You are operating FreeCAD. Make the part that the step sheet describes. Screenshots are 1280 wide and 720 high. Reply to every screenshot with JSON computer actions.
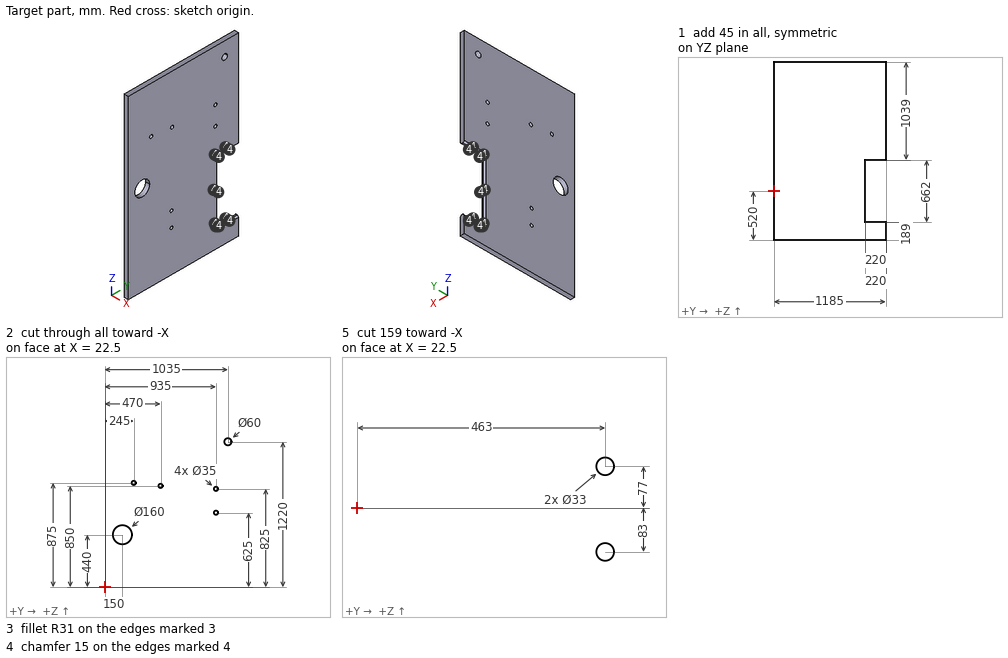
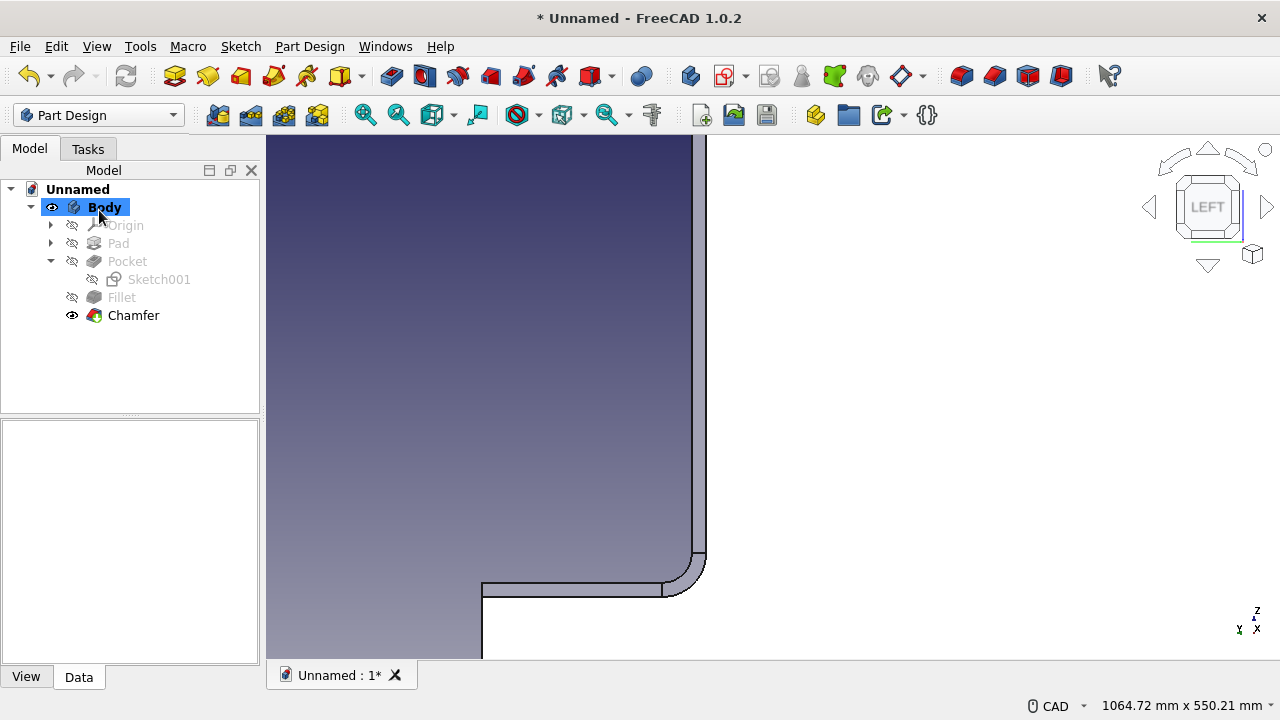
{"action": "left_click", "coordinate": [366, 116]}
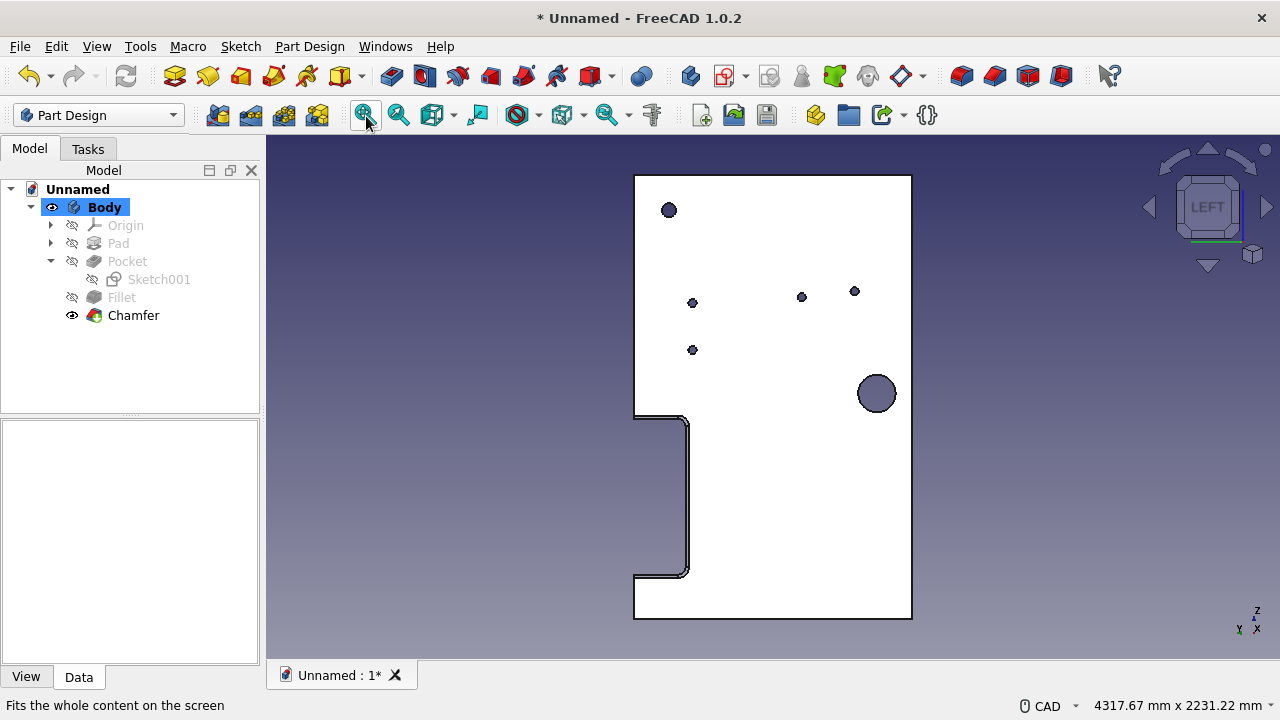
{"action": "key", "text": "0"}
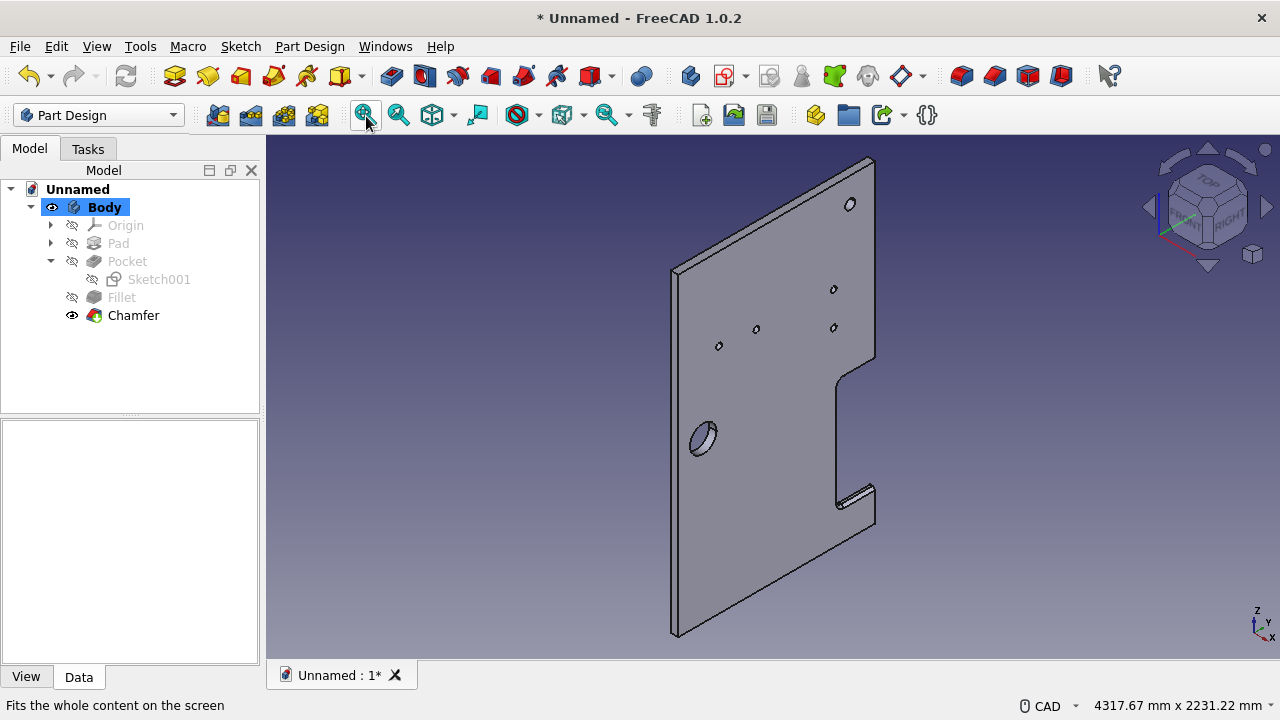
{"action": "left_click", "coordinate": [749, 518]}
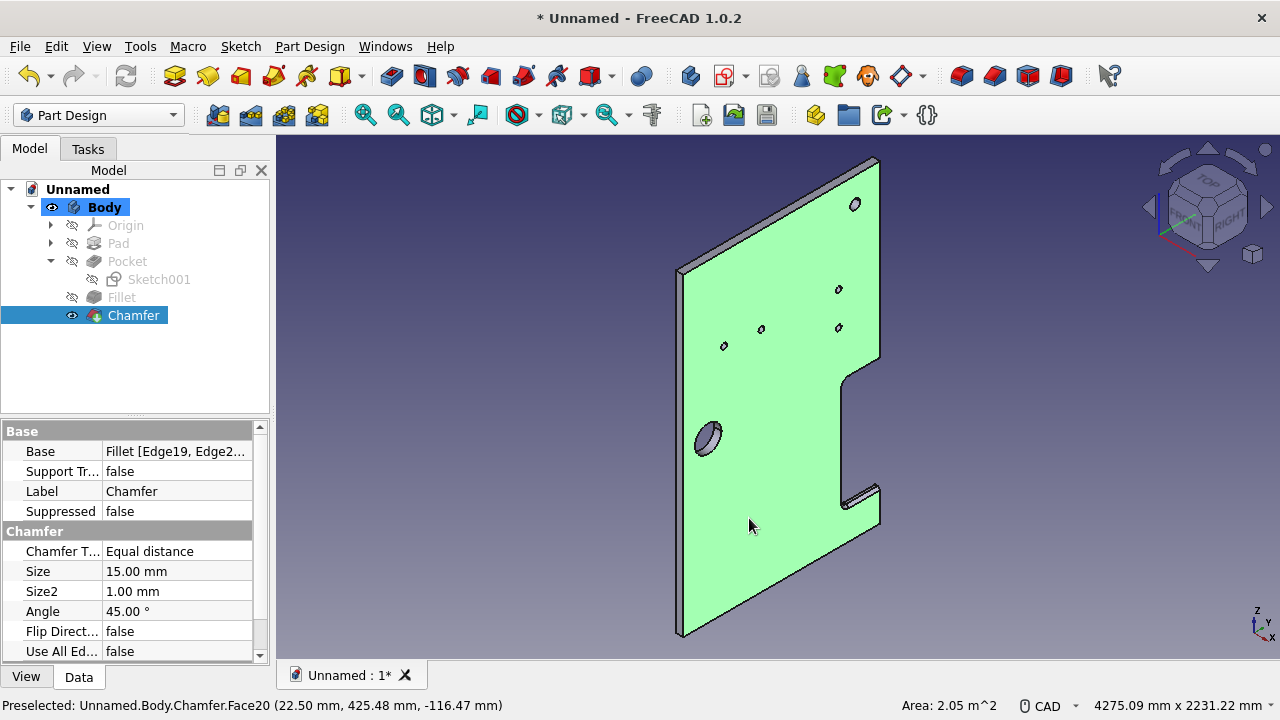
{"action": "left_click", "coordinate": [724, 76]}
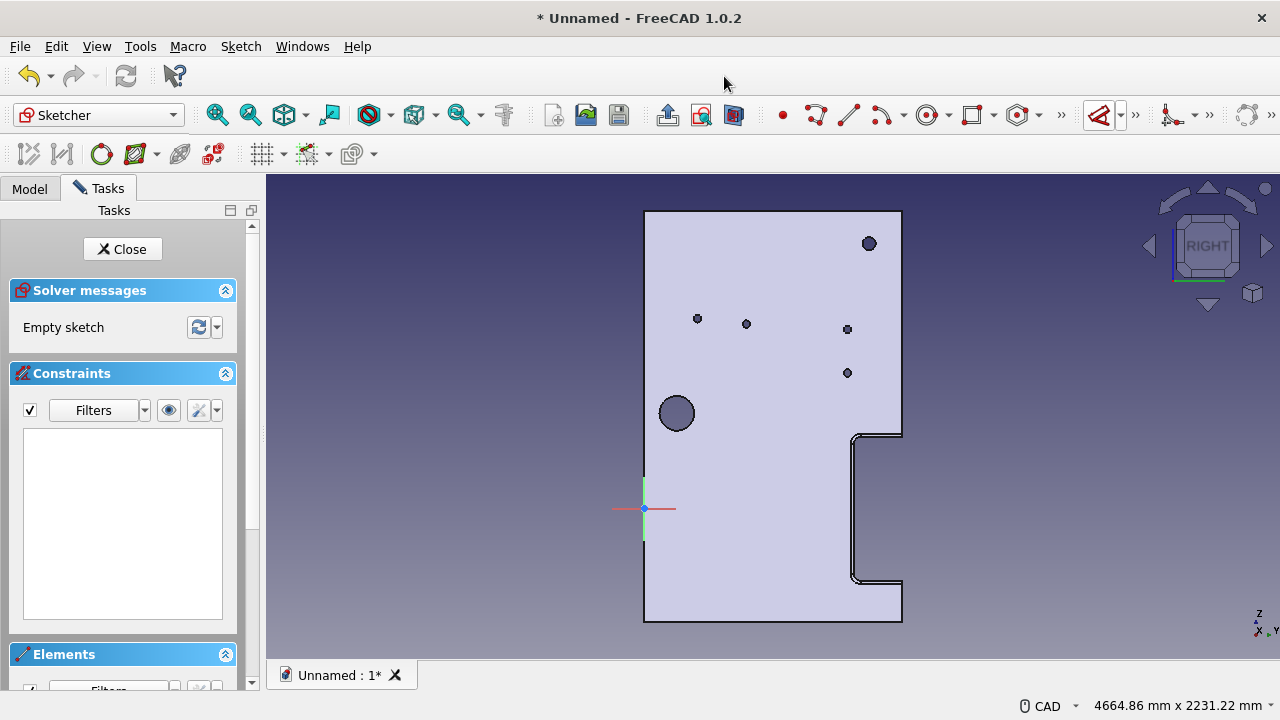
{"action": "scroll", "coordinate": [695, 528], "scroll_direction": "up", "scroll_amount": 9}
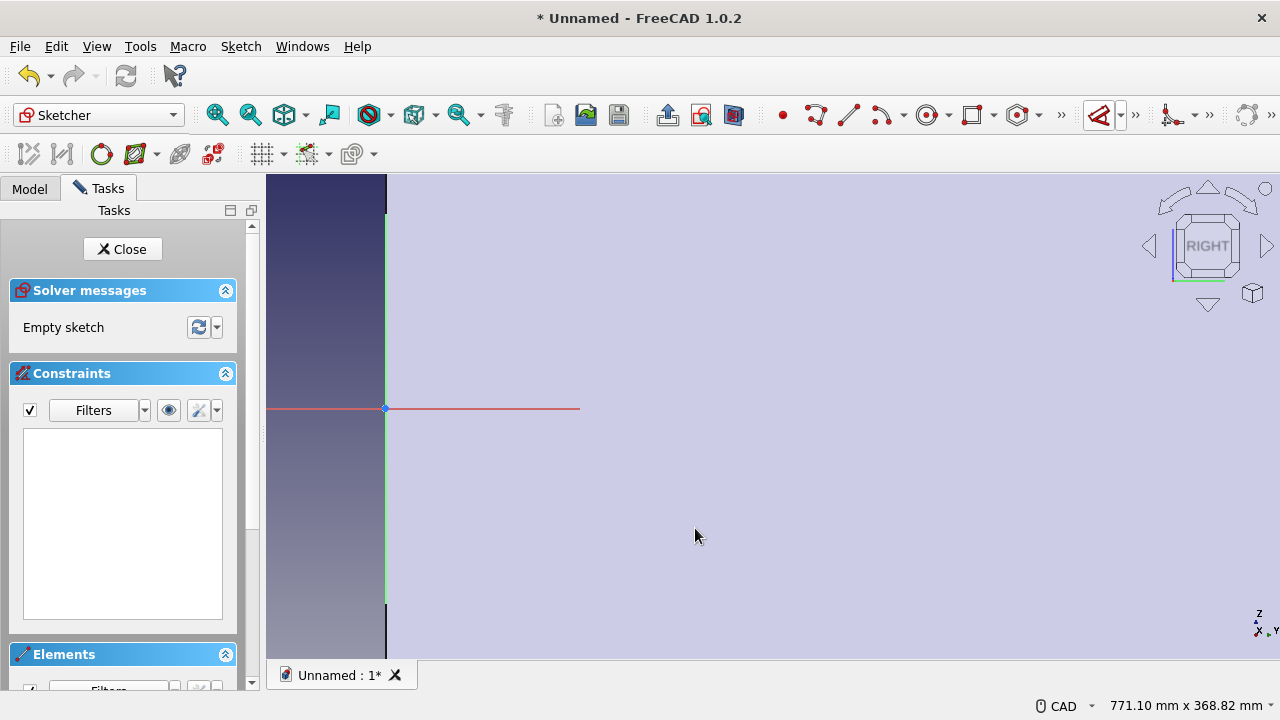
{"action": "left_click", "coordinate": [926, 116]}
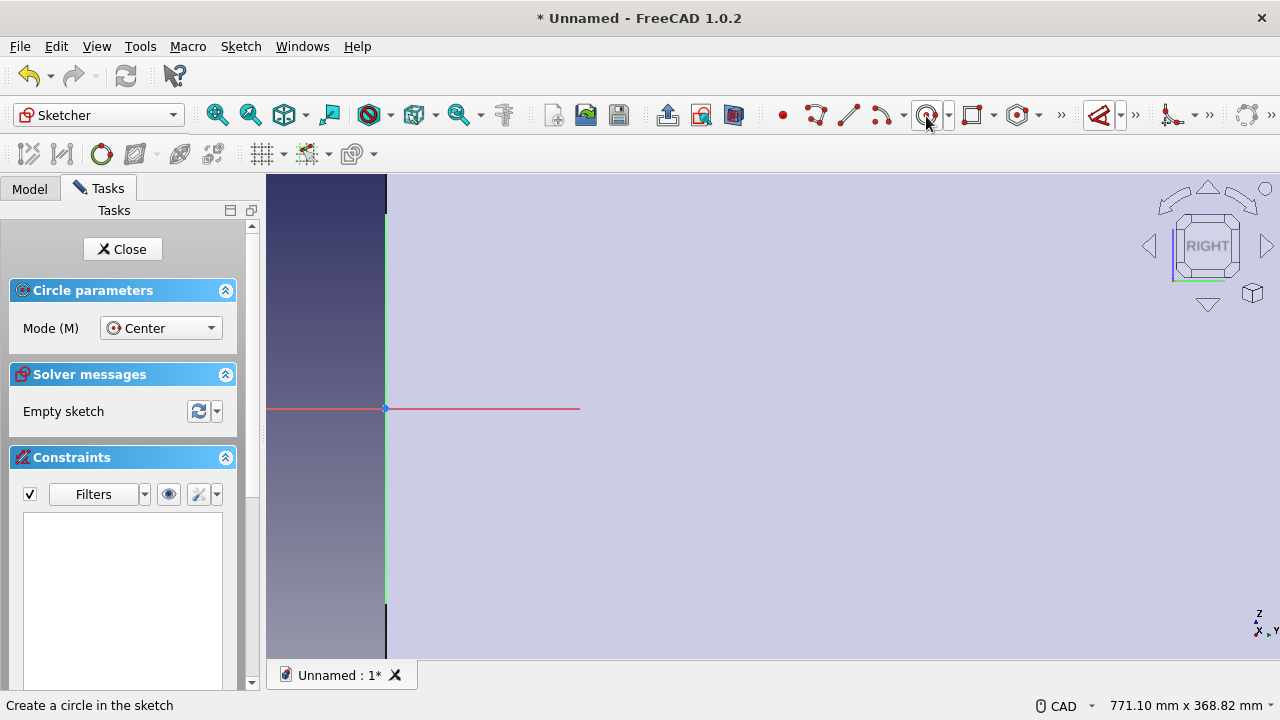
{"action": "left_click", "coordinate": [994, 307]}
{"action": "left_click", "coordinate": [1010, 292]}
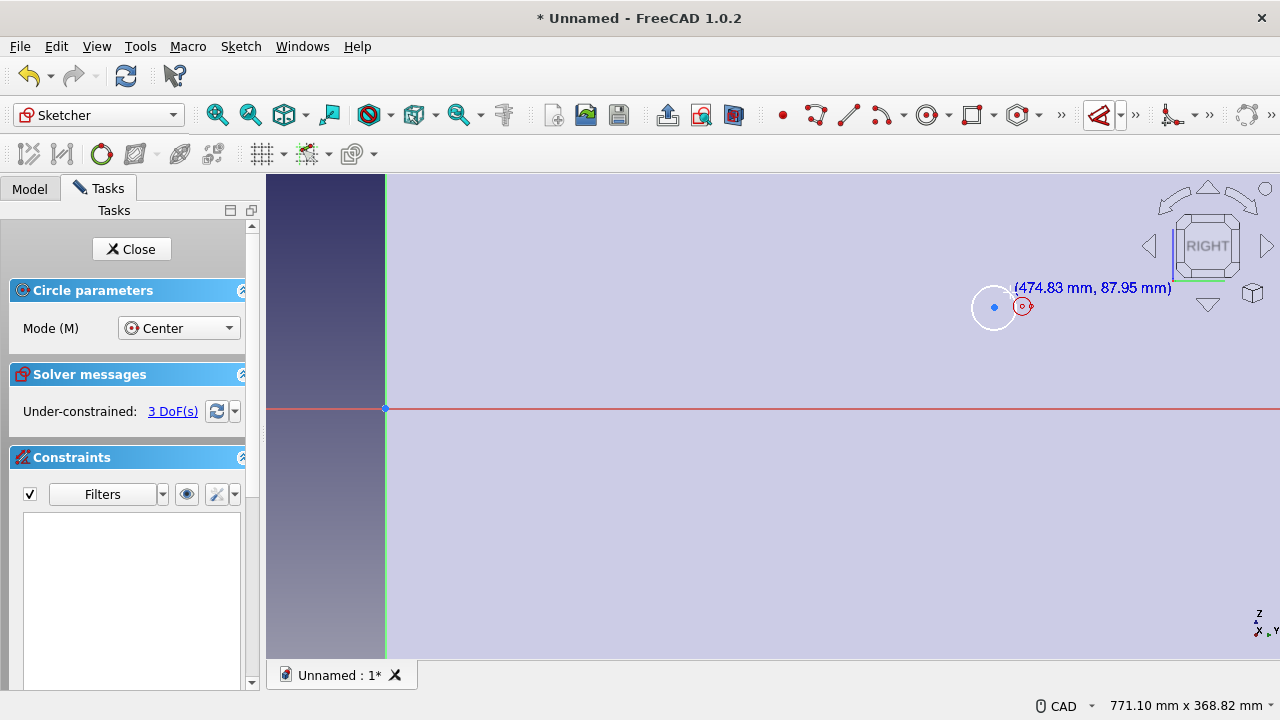
{"action": "left_click", "coordinate": [994, 518]}
{"action": "left_click", "coordinate": [1010, 502]}
{"action": "key", "text": "Escape"}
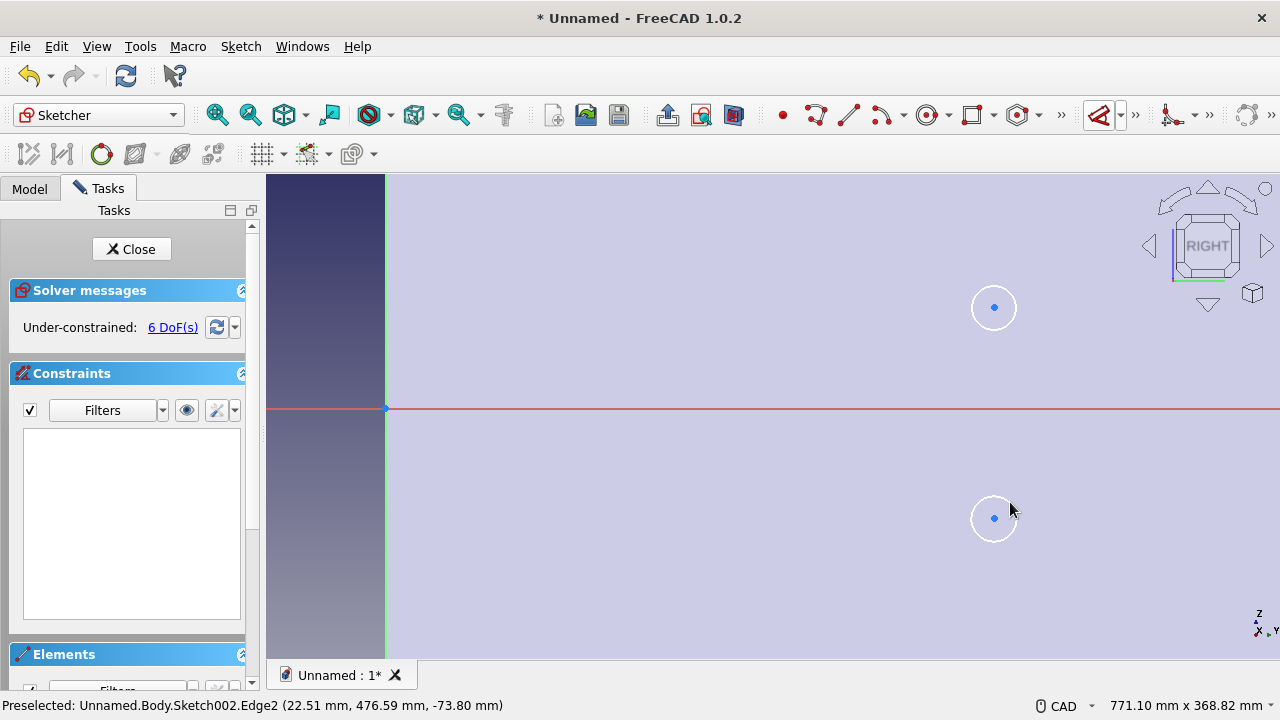
{"action": "left_click", "coordinate": [1009, 292]}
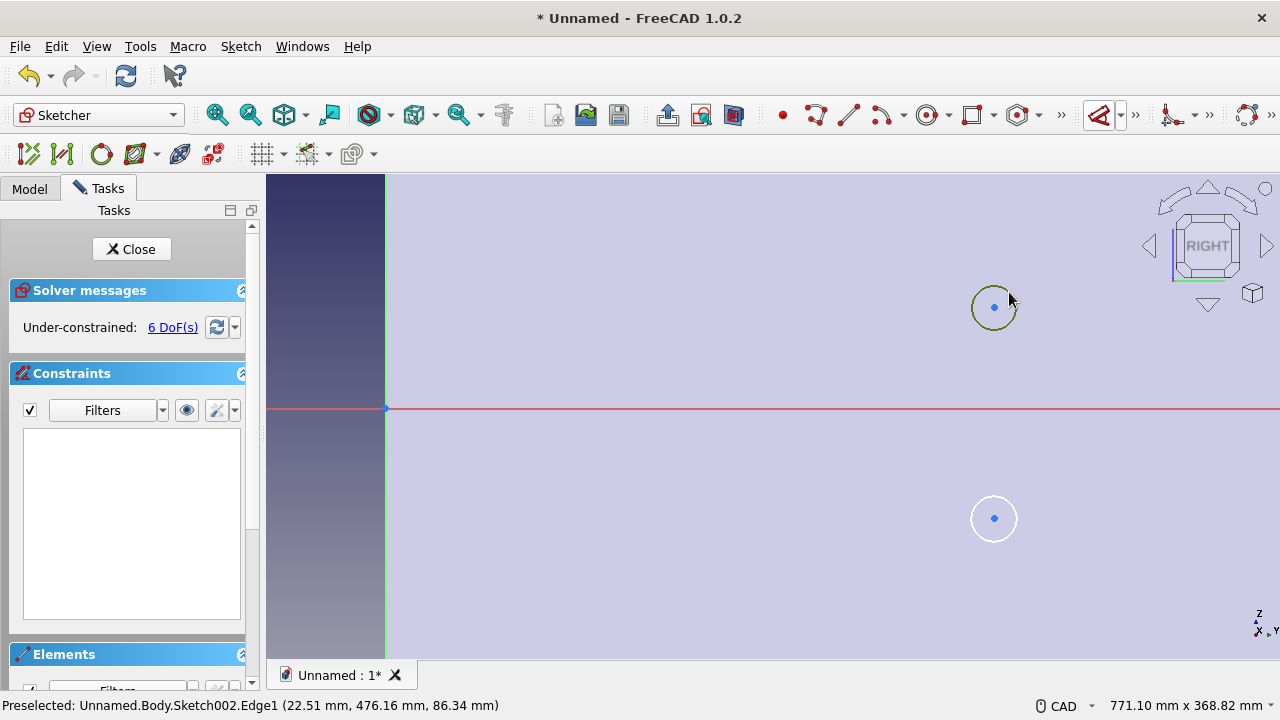
{"action": "left_click", "coordinate": [1010, 503]}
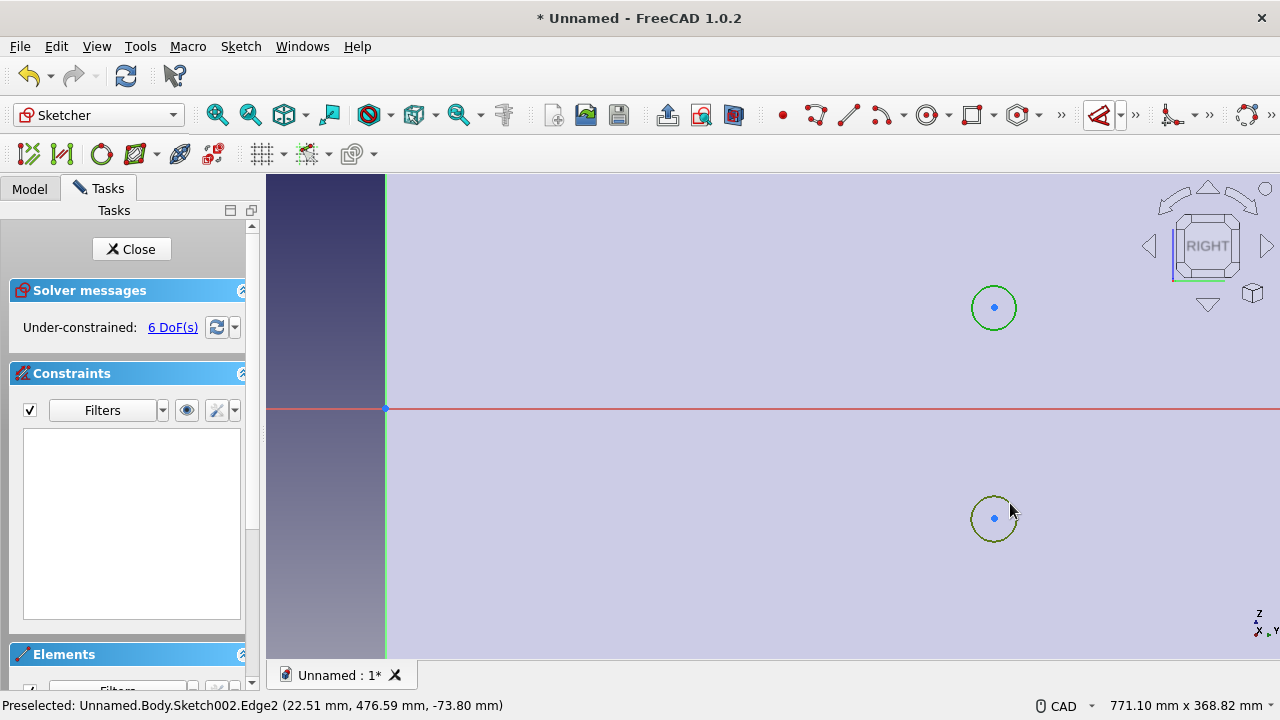
{"action": "key", "text": "e"}